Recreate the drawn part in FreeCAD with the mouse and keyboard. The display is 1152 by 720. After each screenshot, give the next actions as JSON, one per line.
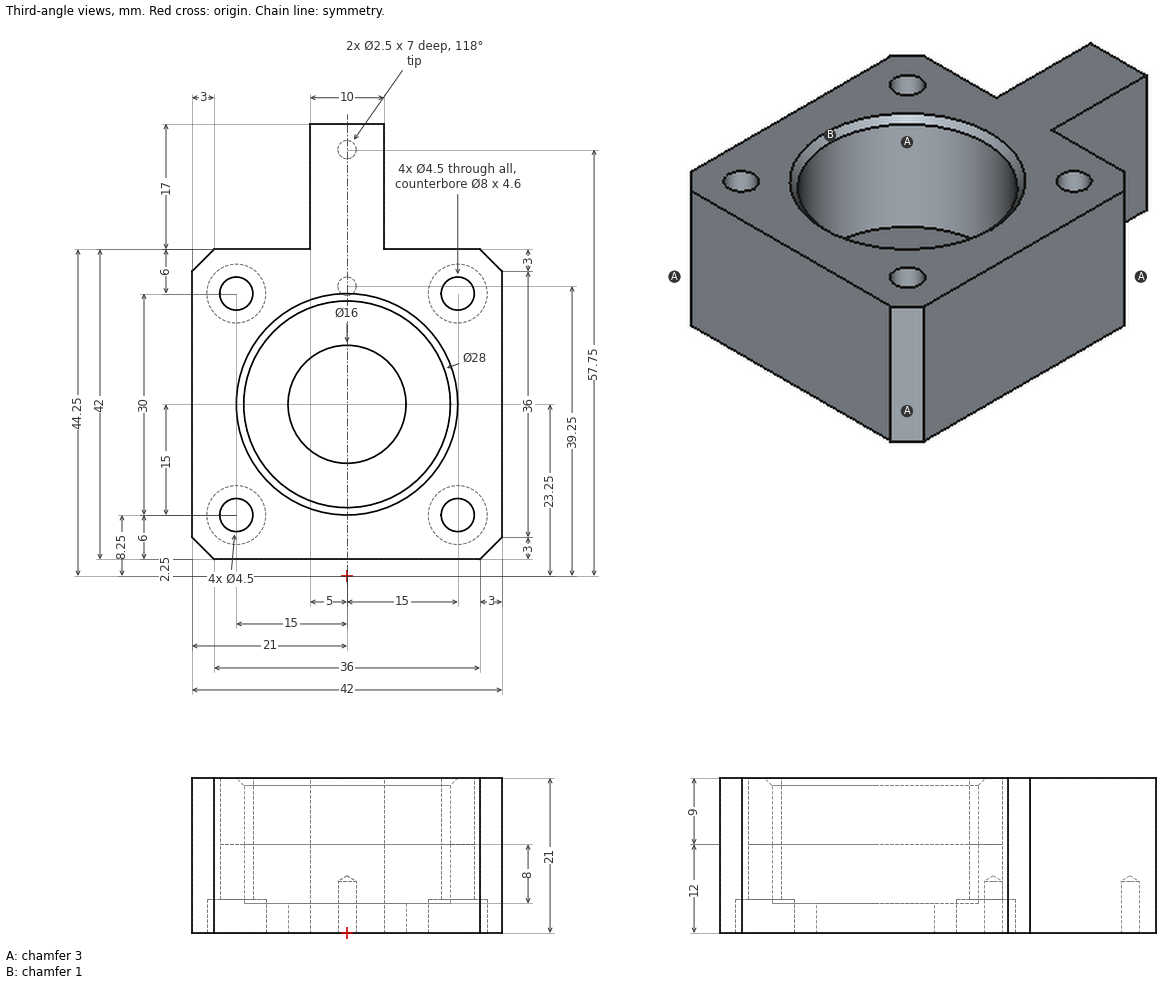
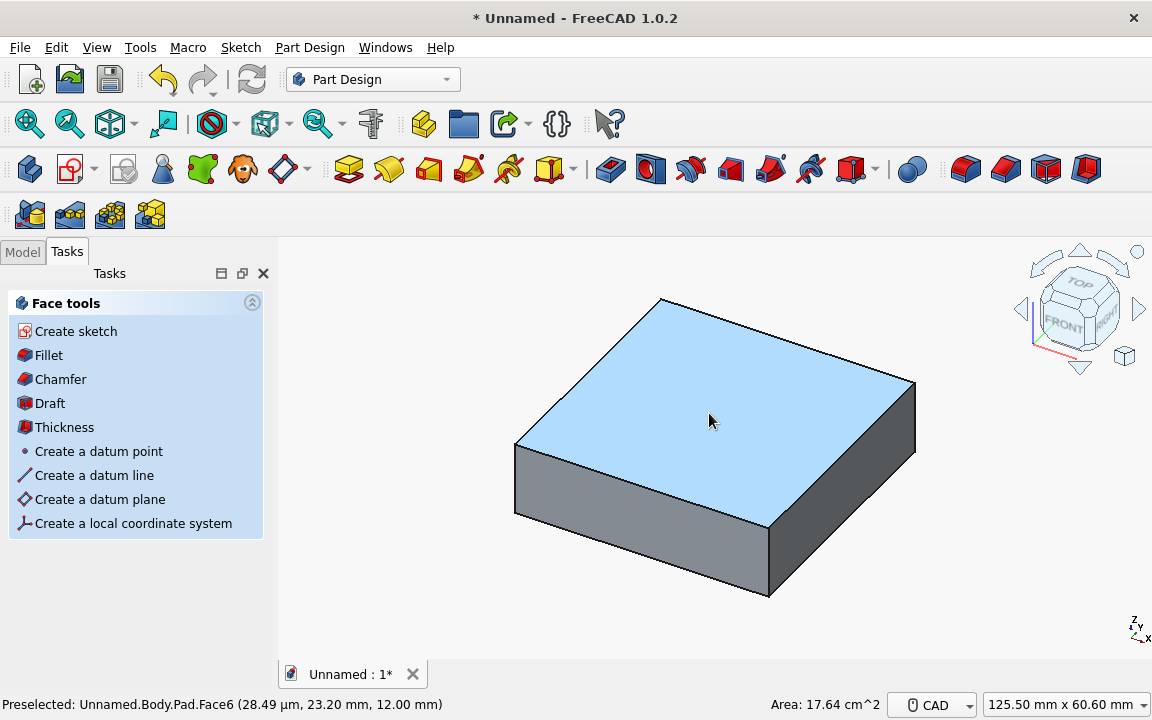
{"action": "left_click", "coordinate": [70, 170]}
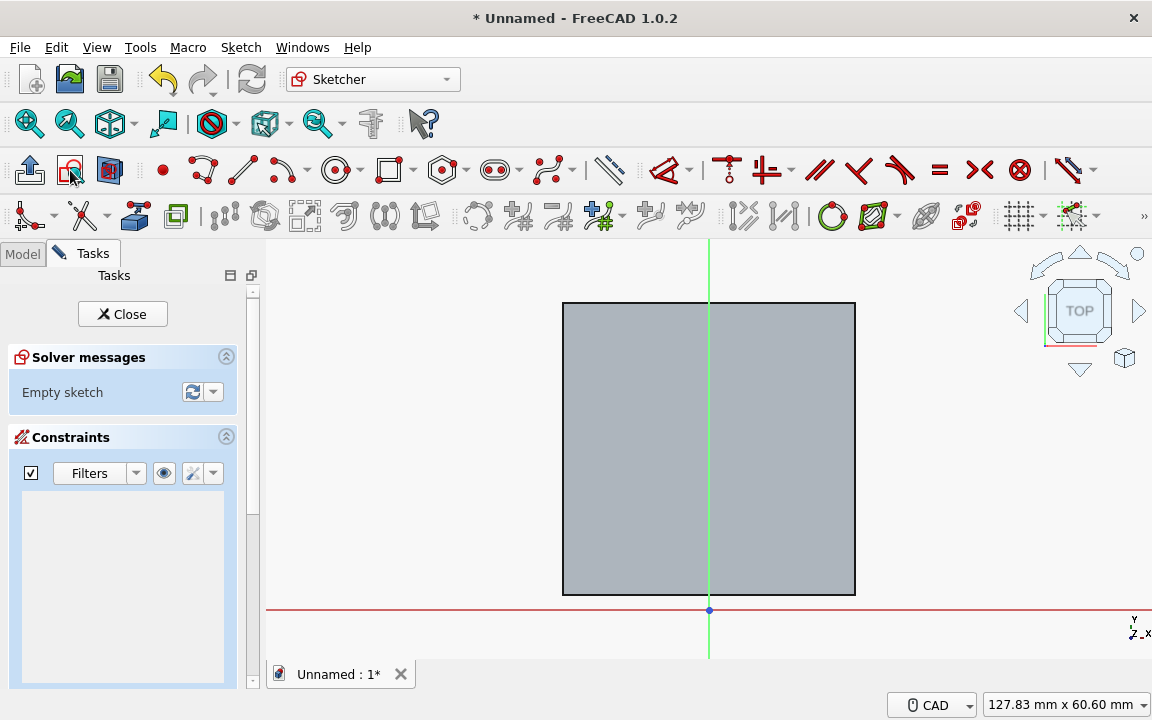
{"action": "scroll", "coordinate": [331, 304], "scroll_direction": "down", "scroll_amount": 1}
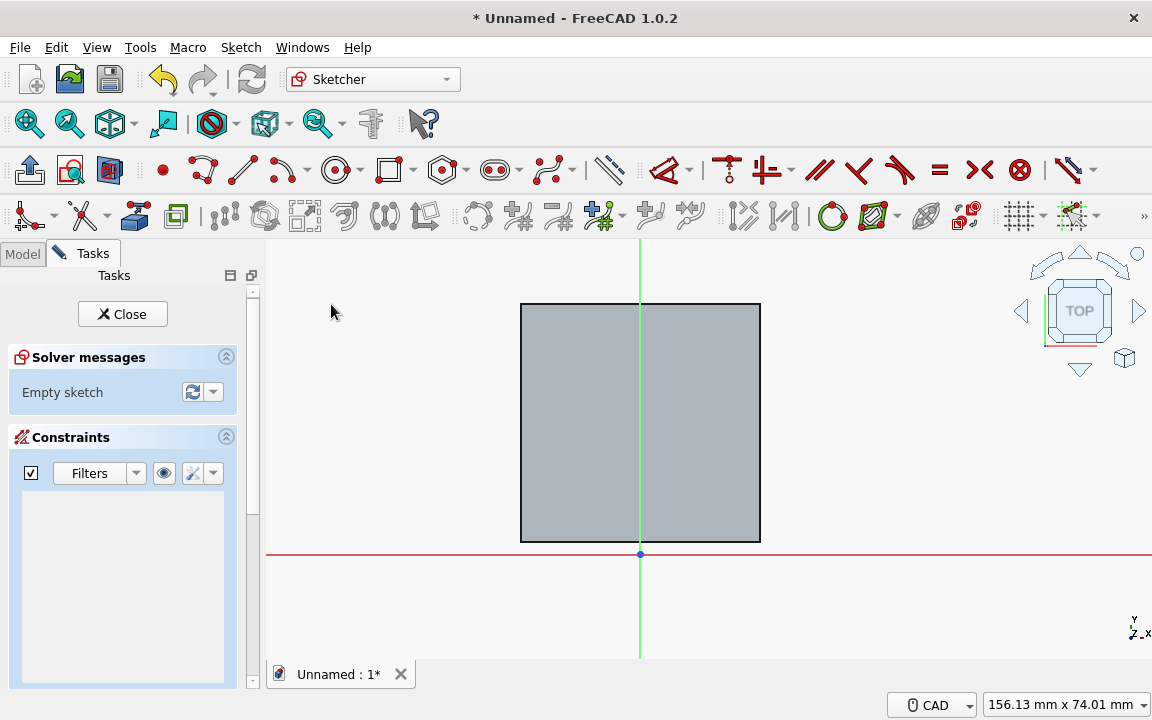
{"action": "left_click", "coordinate": [336, 170]}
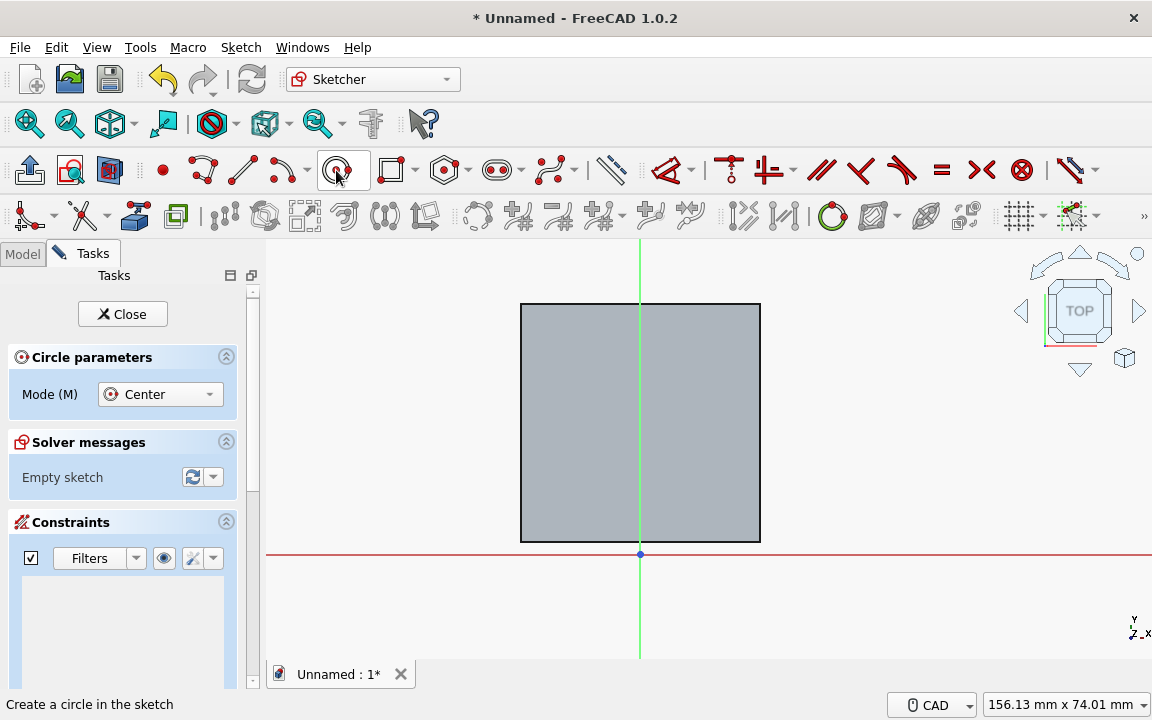
{"action": "left_click", "coordinate": [640, 423]}
{"action": "left_click", "coordinate": [697, 367]}
{"action": "key", "text": "Escape"}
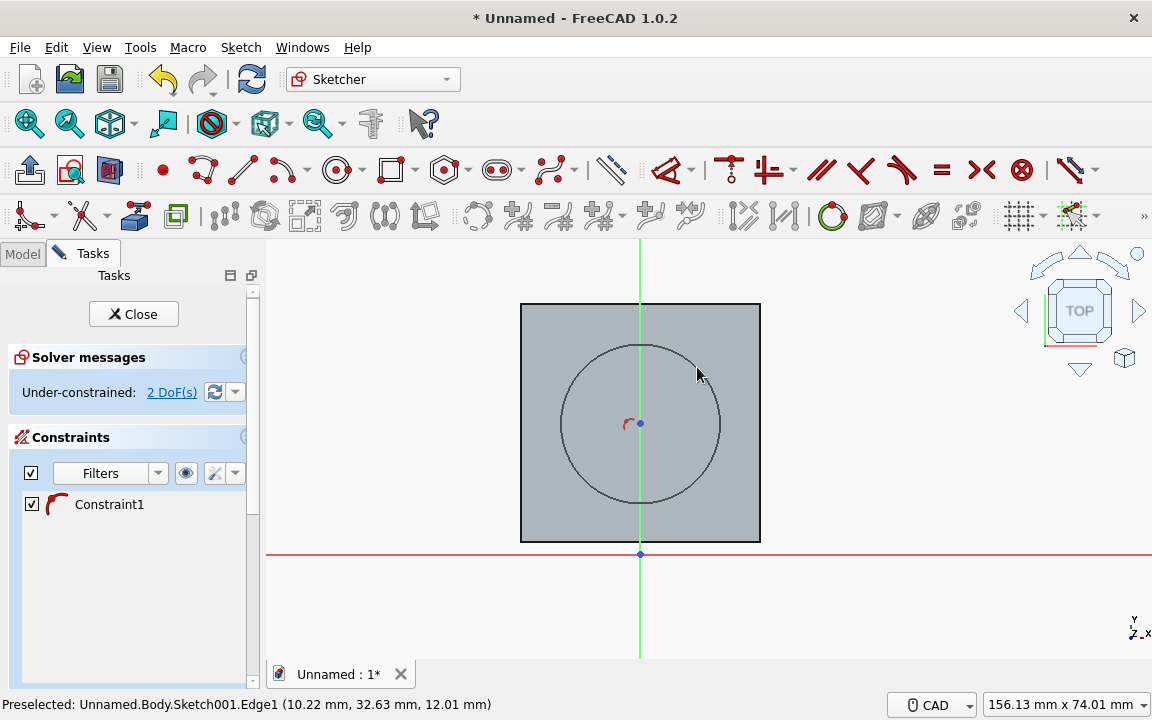
{"action": "left_click", "coordinate": [666, 170]}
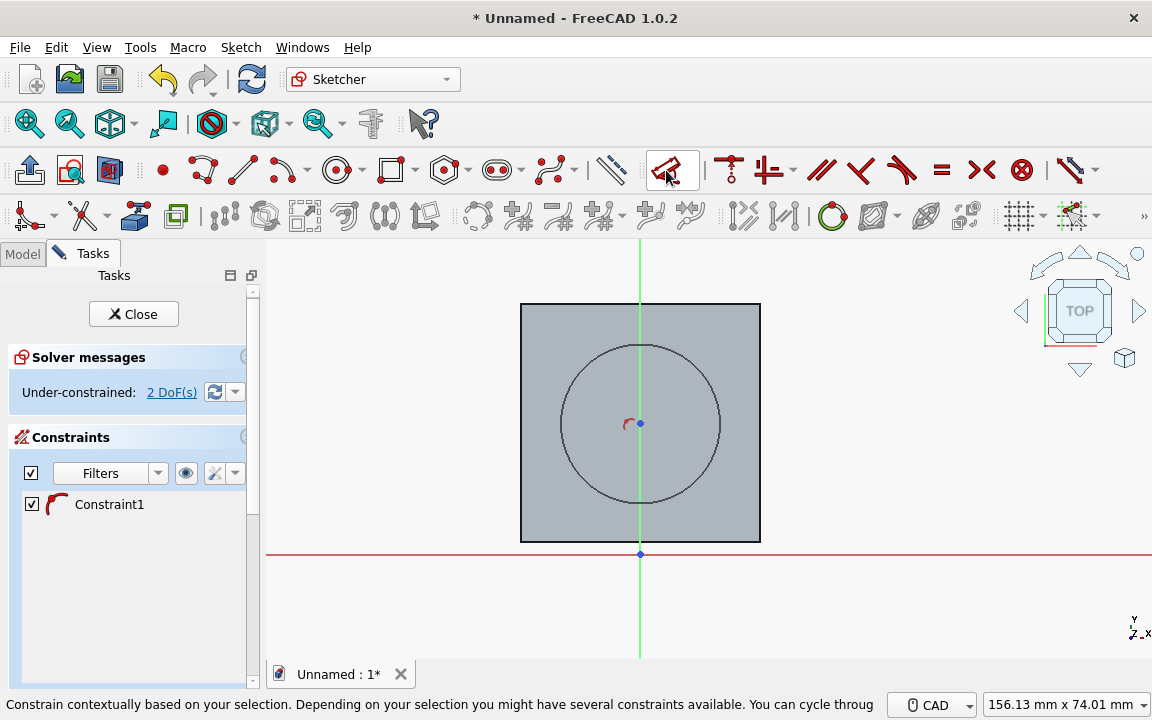
{"action": "left_click", "coordinate": [697, 368]}
{"action": "left_click", "coordinate": [720, 345]}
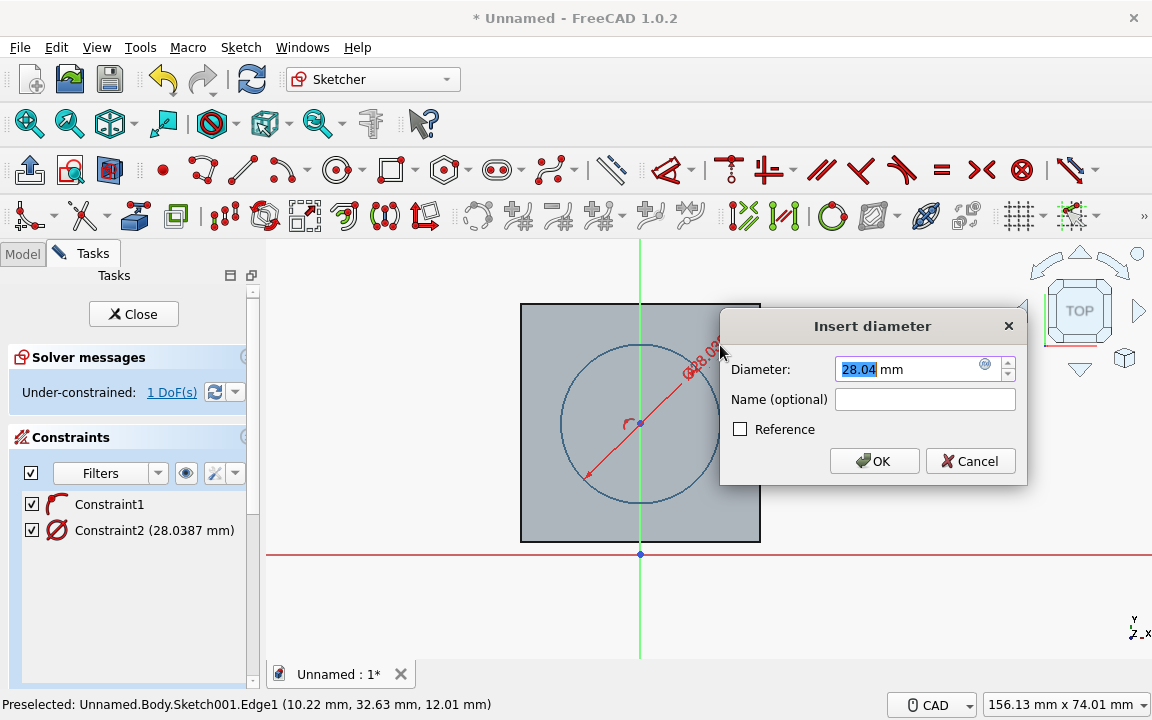
{"action": "type", "text": "28"}
{"action": "key", "text": "Return"}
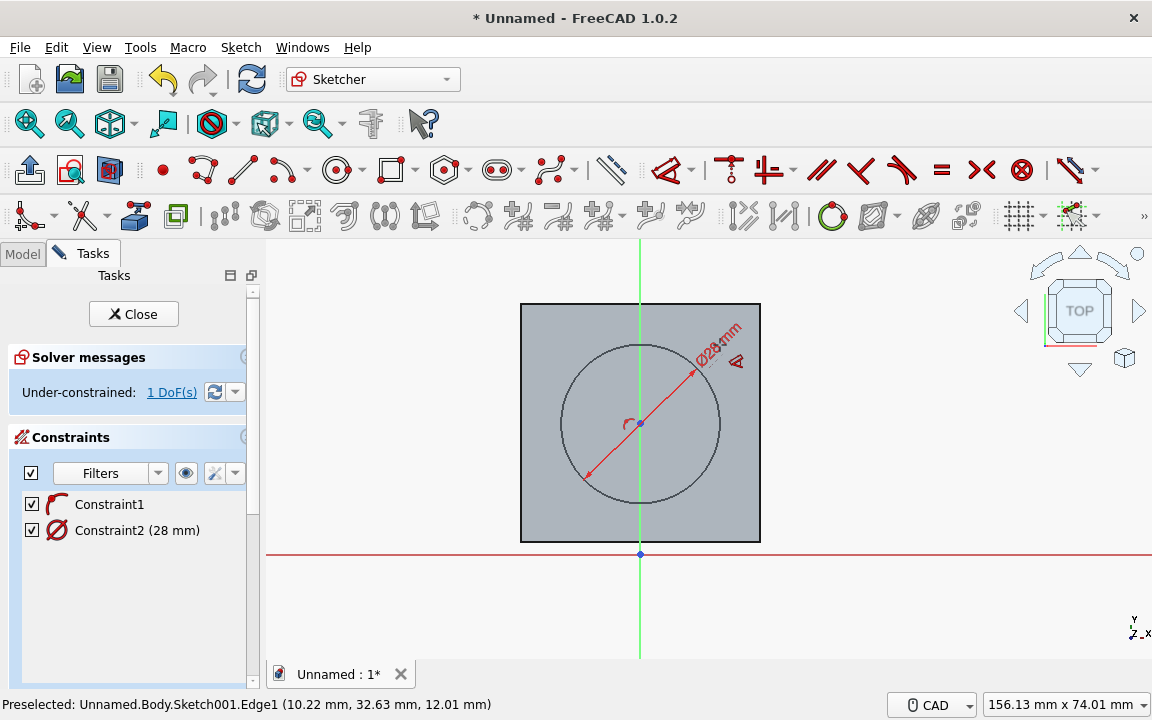
{"action": "left_click", "coordinate": [640, 424]}
{"action": "left_click", "coordinate": [674, 459]}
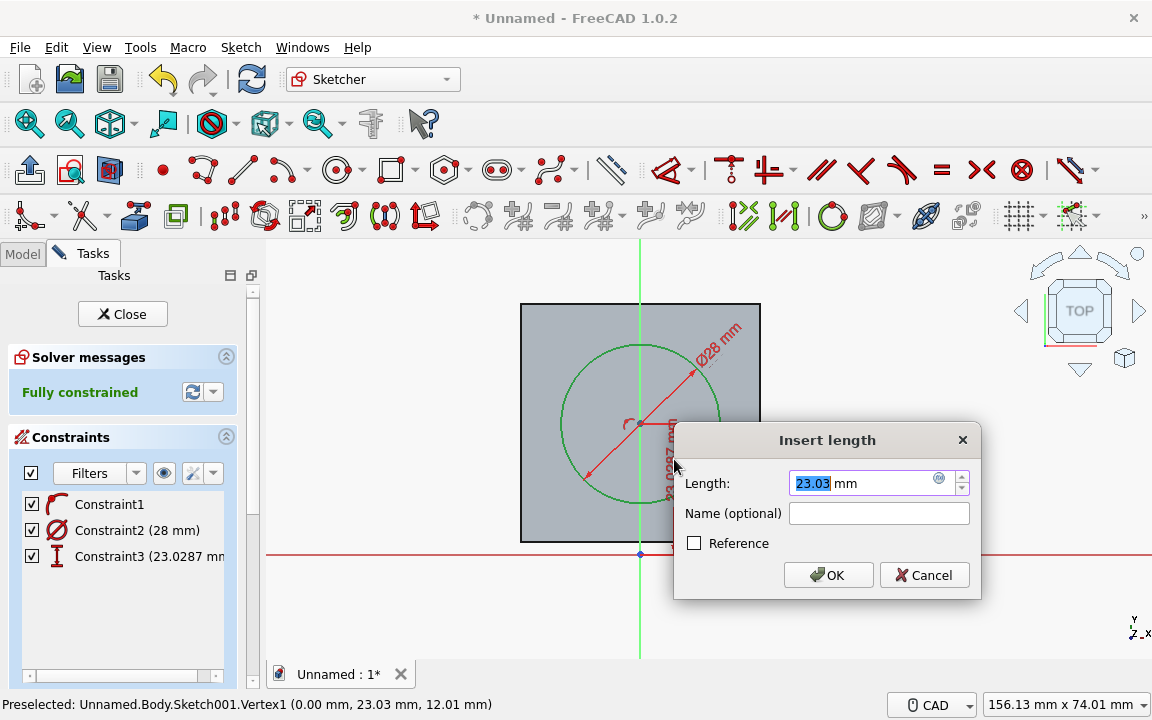
{"action": "type", "text": "23.25"}
{"action": "key", "text": "Return"}
{"action": "key", "text": "Escape"}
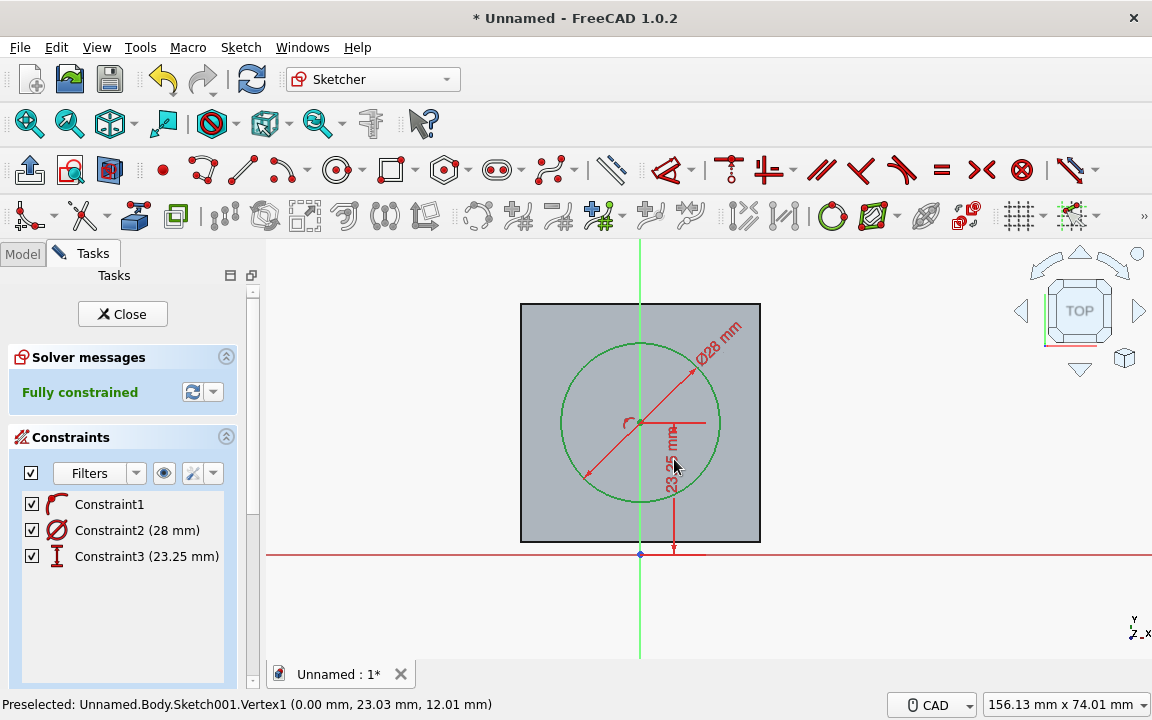
{"action": "left_click", "coordinate": [123, 314]}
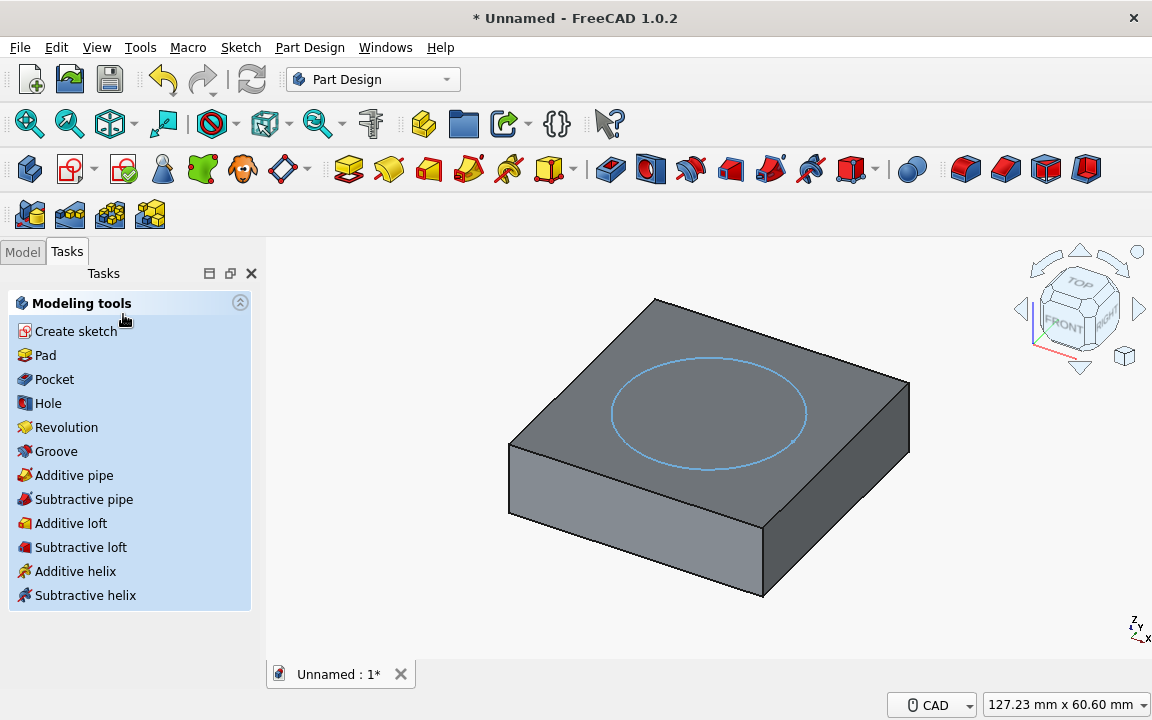
{"action": "left_click", "coordinate": [612, 170]}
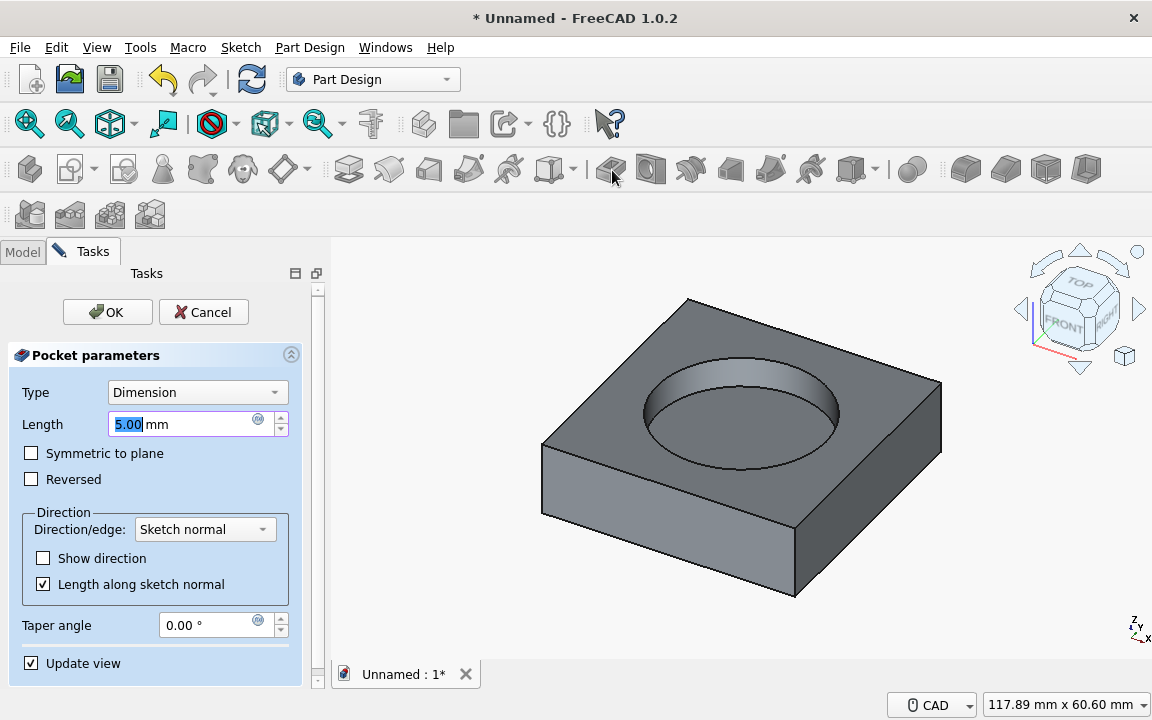
{"action": "type", "text": "8"}
{"action": "key", "text": "Tab"}